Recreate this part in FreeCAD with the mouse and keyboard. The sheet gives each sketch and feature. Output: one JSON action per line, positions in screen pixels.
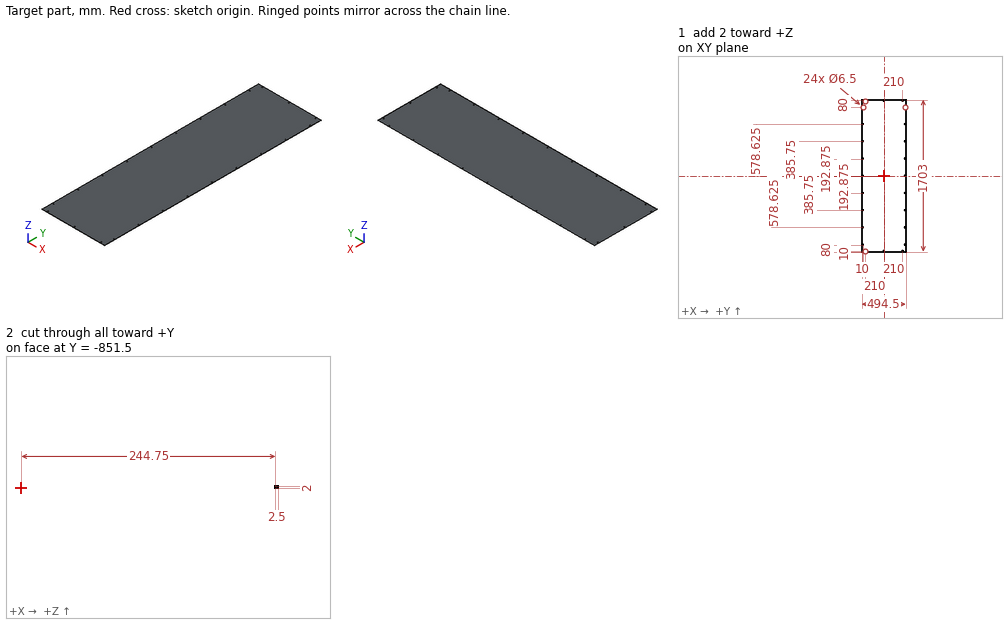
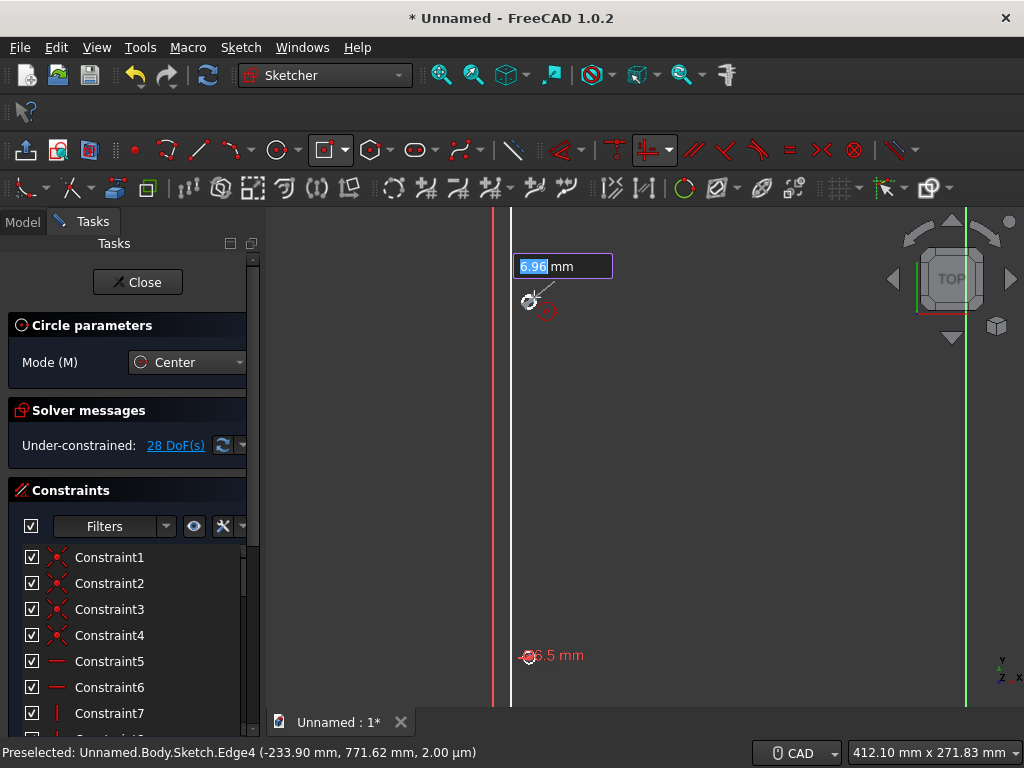
{"action": "type", "text": "6.5"}
{"action": "key", "text": "Return"}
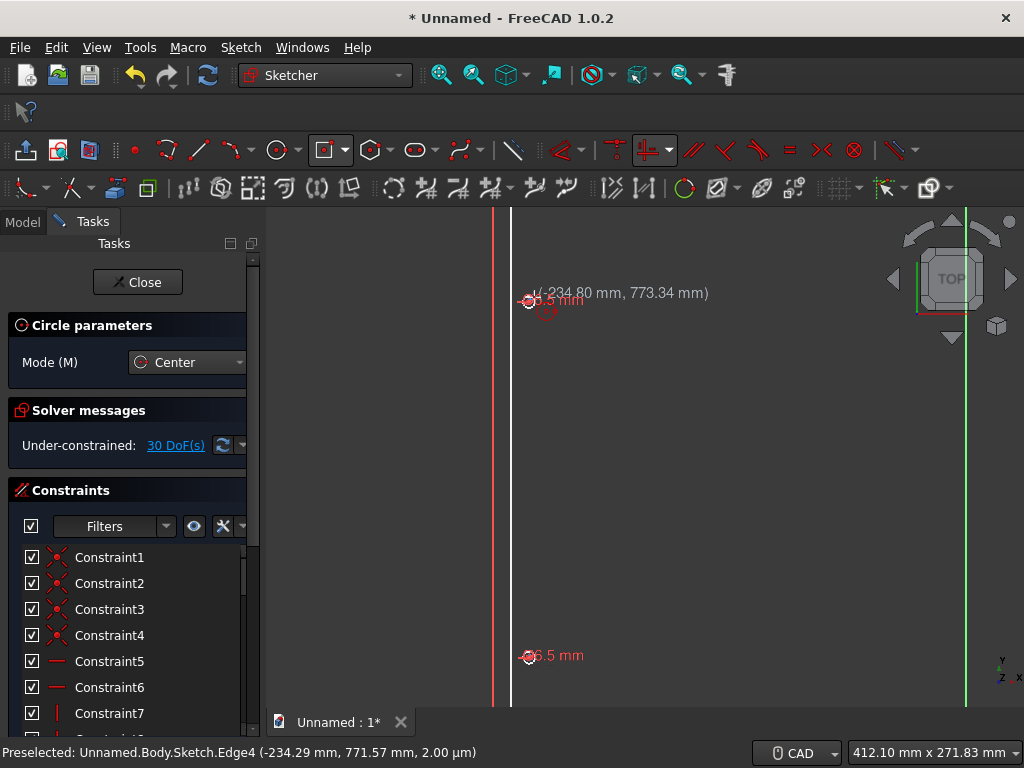
{"action": "scroll", "coordinate": [538, 331], "scroll_direction": "down", "scroll_amount": 12}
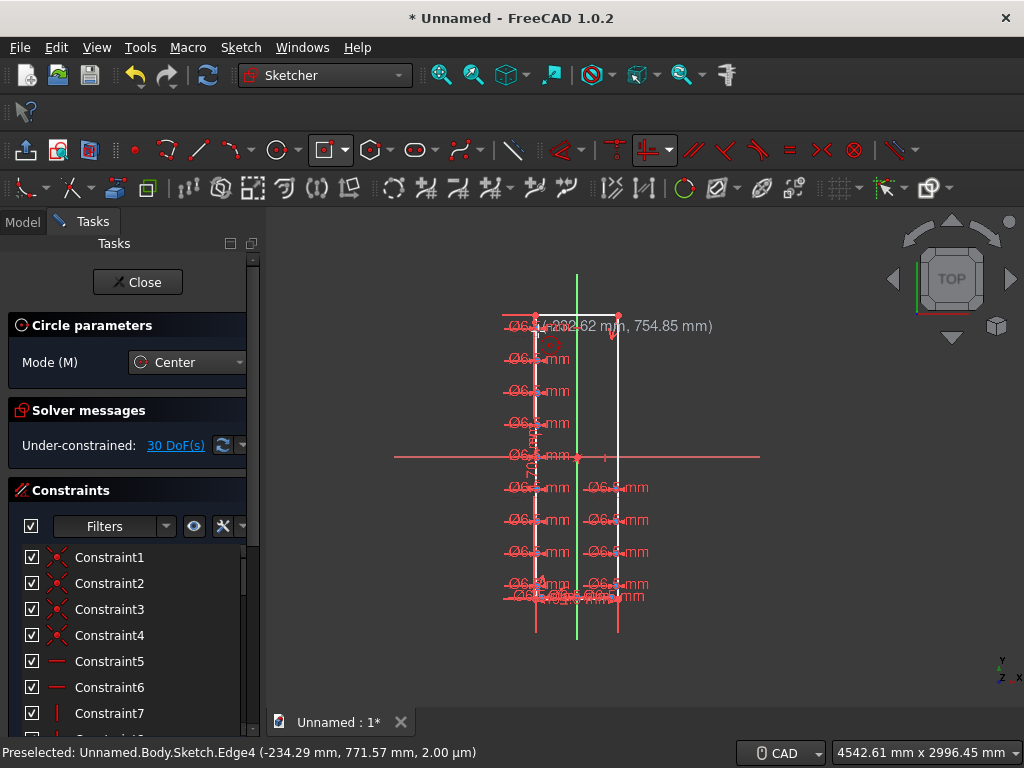
{"action": "scroll", "coordinate": [542, 317], "scroll_direction": "up", "scroll_amount": 19}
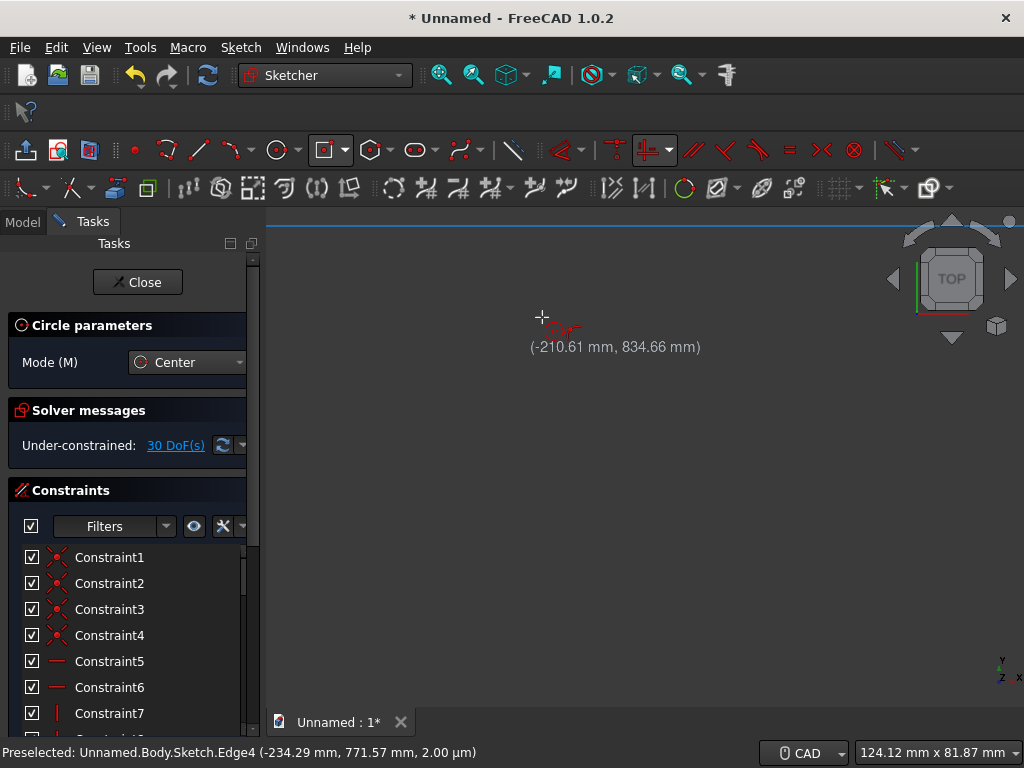
{"action": "scroll", "coordinate": [534, 285], "scroll_direction": "down", "scroll_amount": 18}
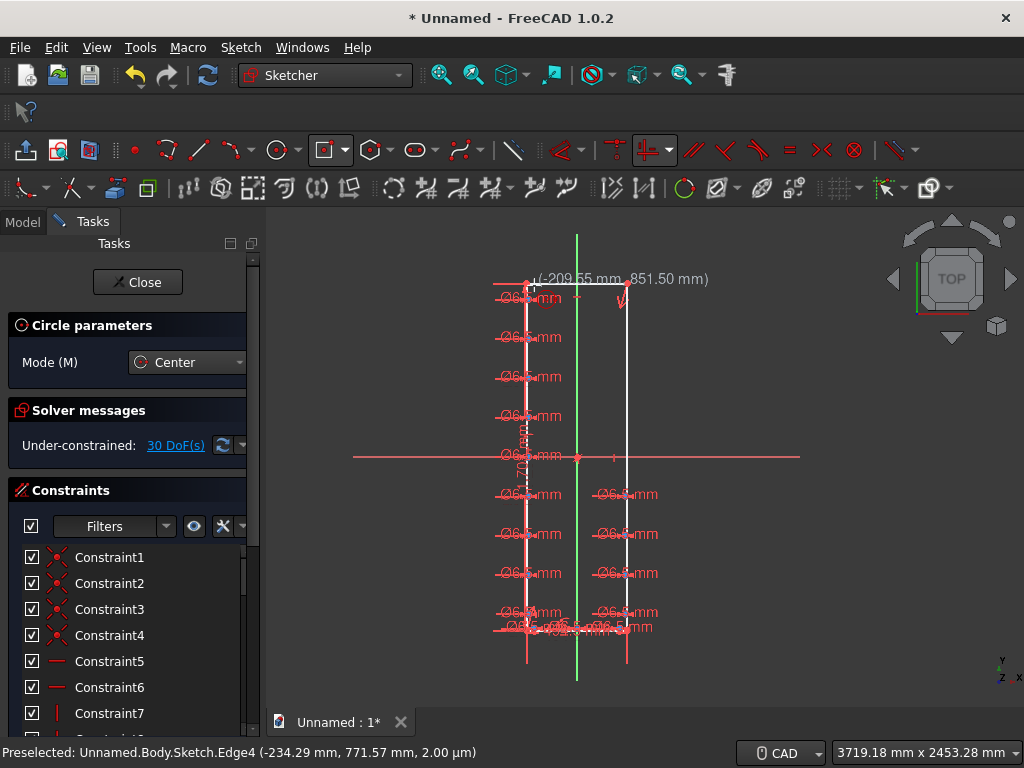
{"action": "scroll", "coordinate": [534, 286], "scroll_direction": "up", "scroll_amount": 11}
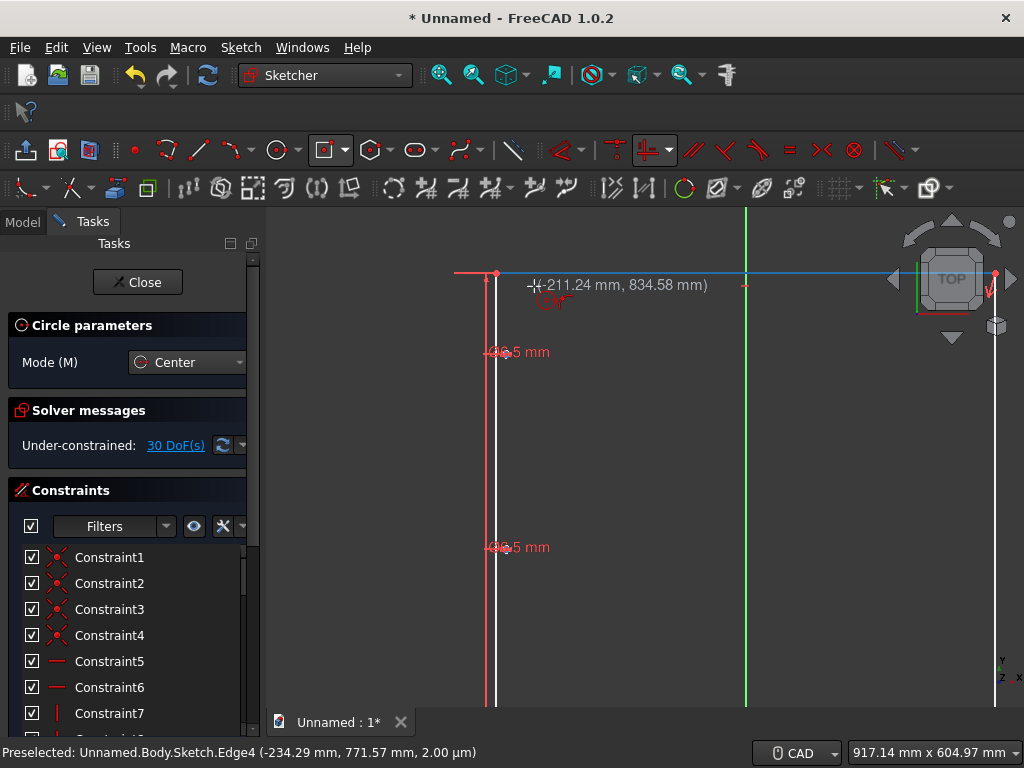
{"action": "left_click", "coordinate": [533, 281]}
{"action": "mouse_move", "coordinate": [538, 277]}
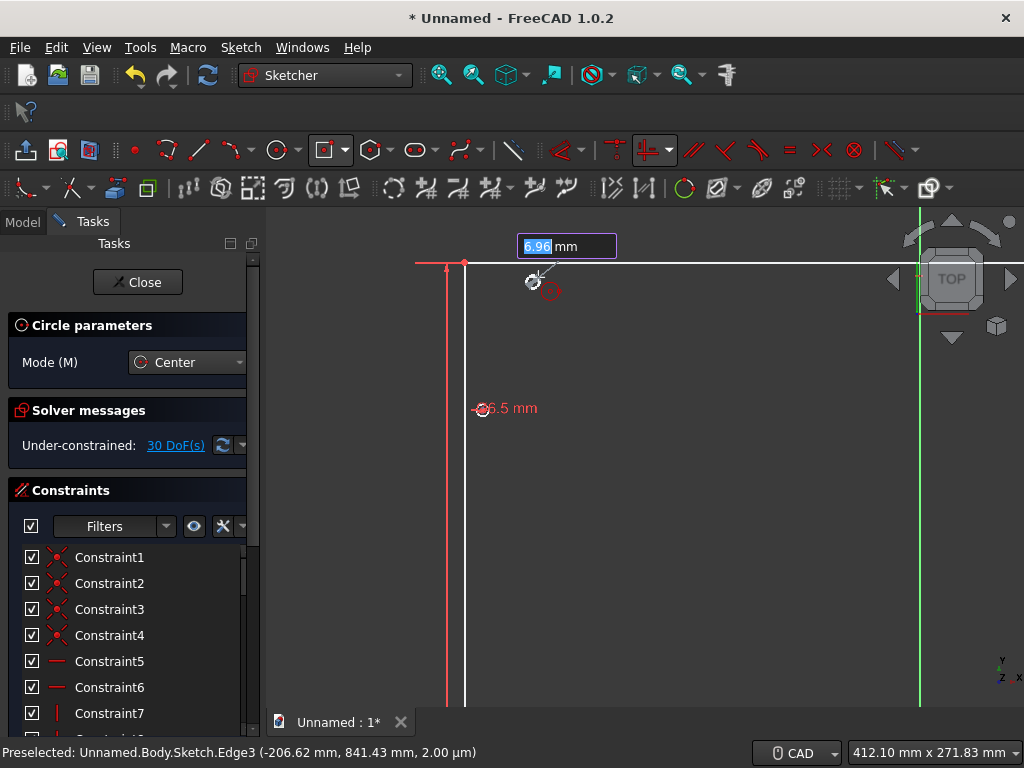
{"action": "type", "text": "6.5"}
{"action": "key", "text": "Return"}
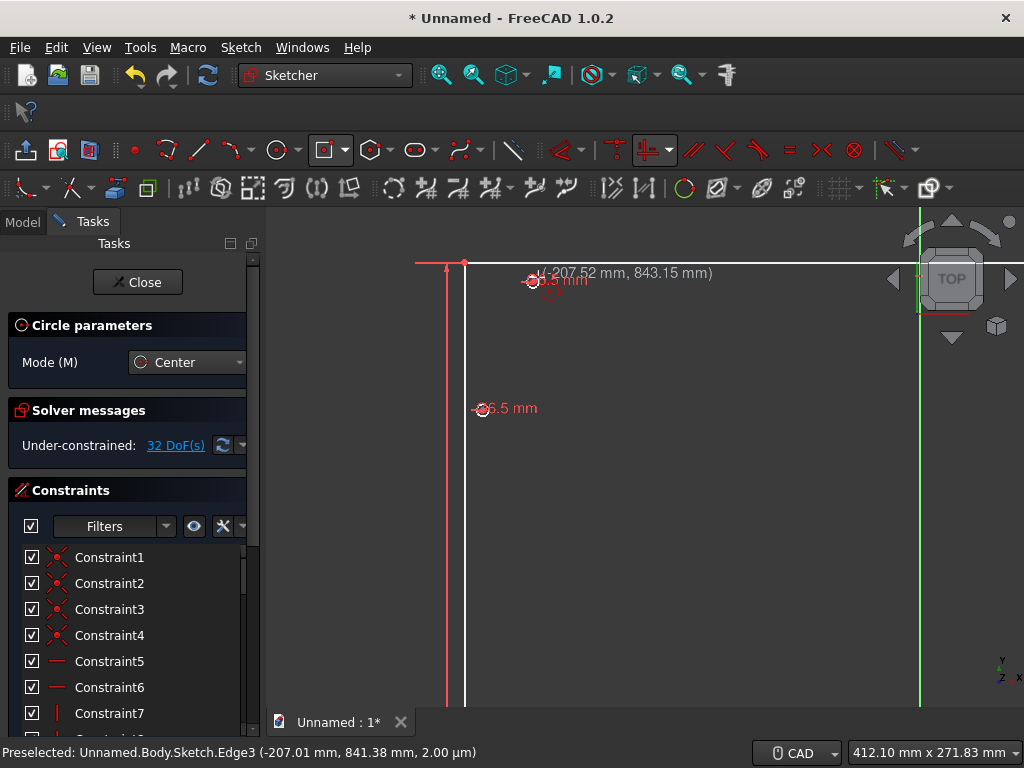
{"action": "scroll", "coordinate": [542, 320], "scroll_direction": "down", "scroll_amount": 12}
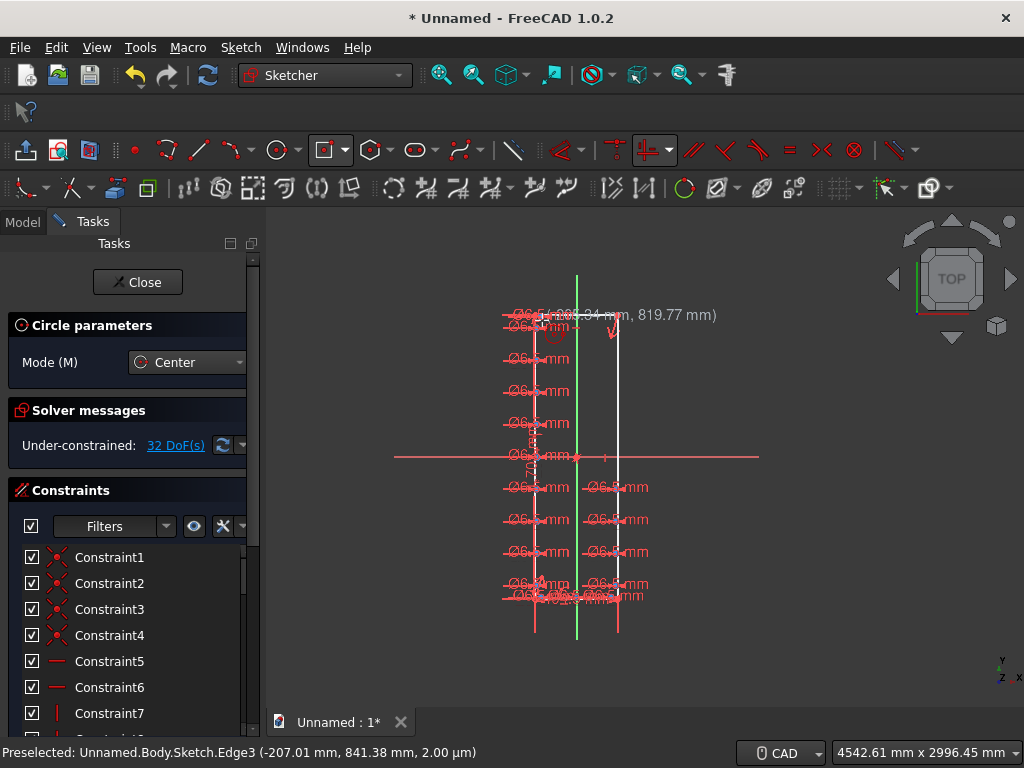
{"action": "scroll", "coordinate": [616, 457], "scroll_direction": "up", "scroll_amount": 19}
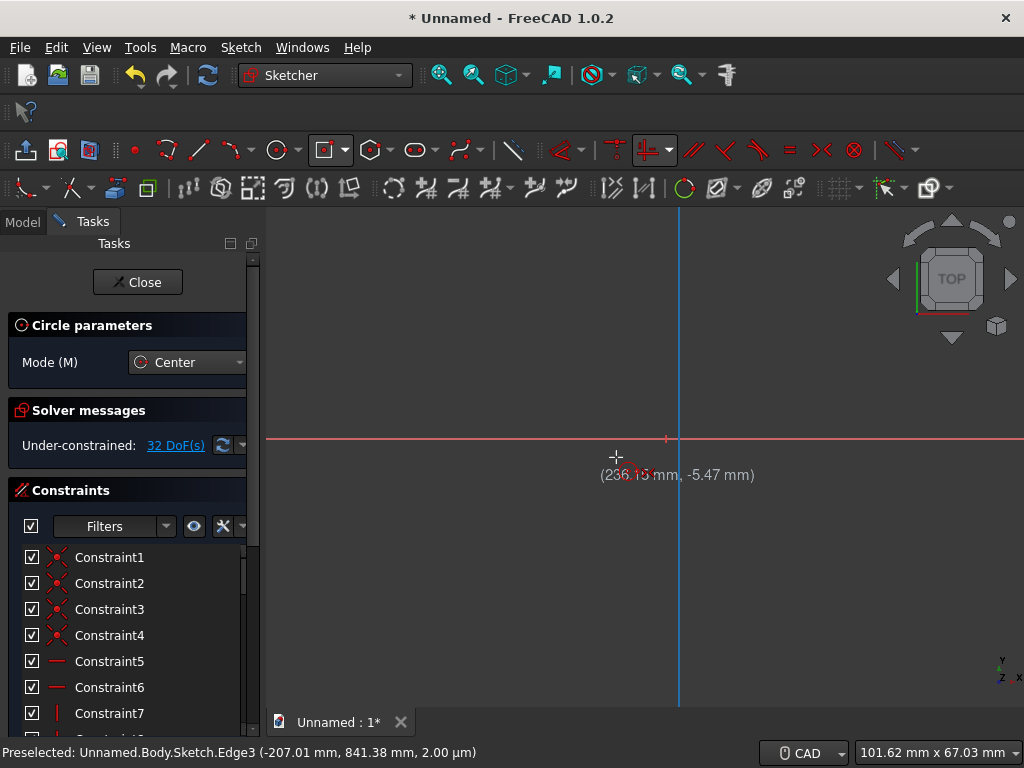
{"action": "scroll", "coordinate": [625, 458], "scroll_direction": "down", "scroll_amount": 18}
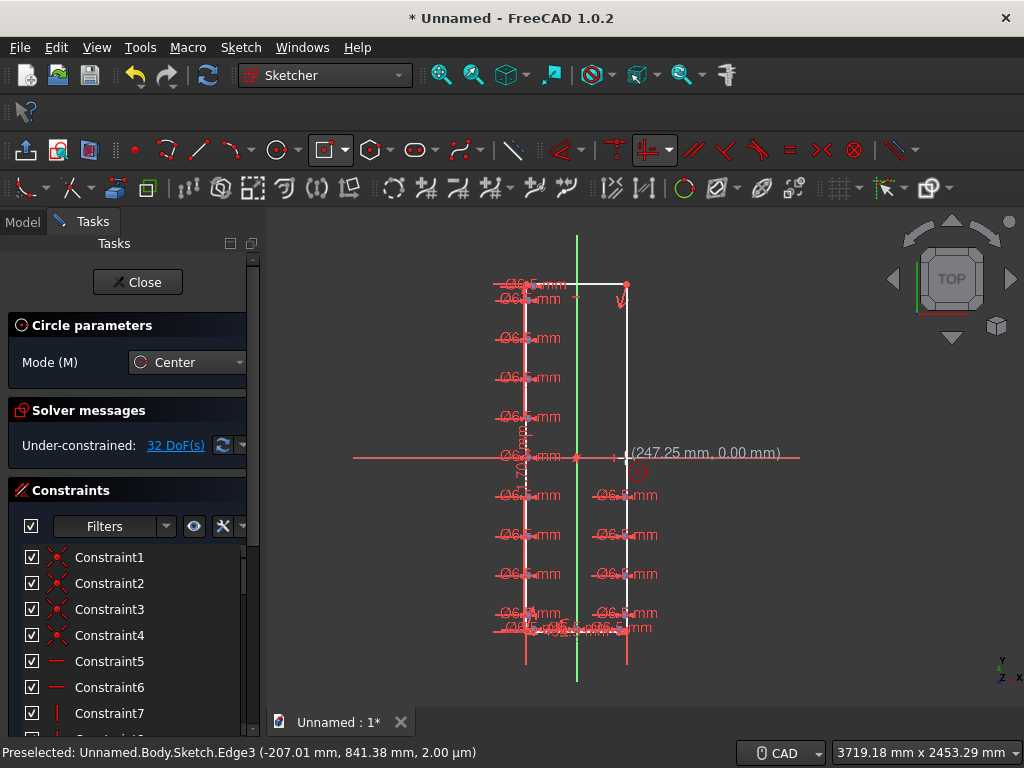
{"action": "scroll", "coordinate": [625, 458], "scroll_direction": "up", "scroll_amount": 11}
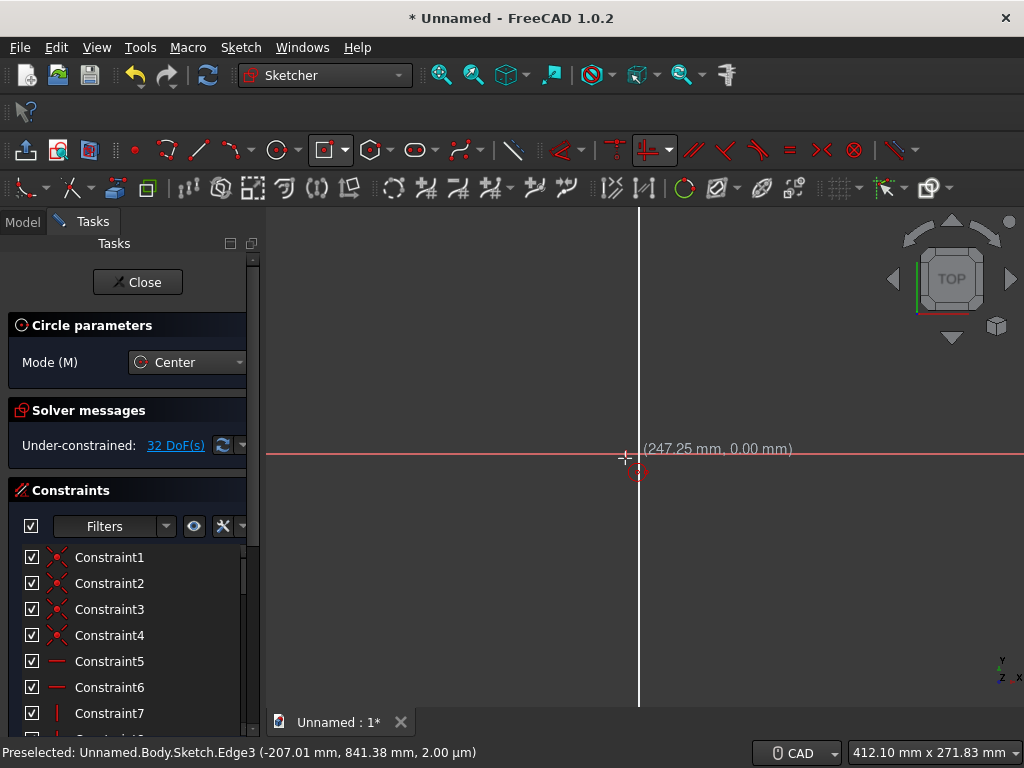
{"action": "left_click", "coordinate": [620, 454]}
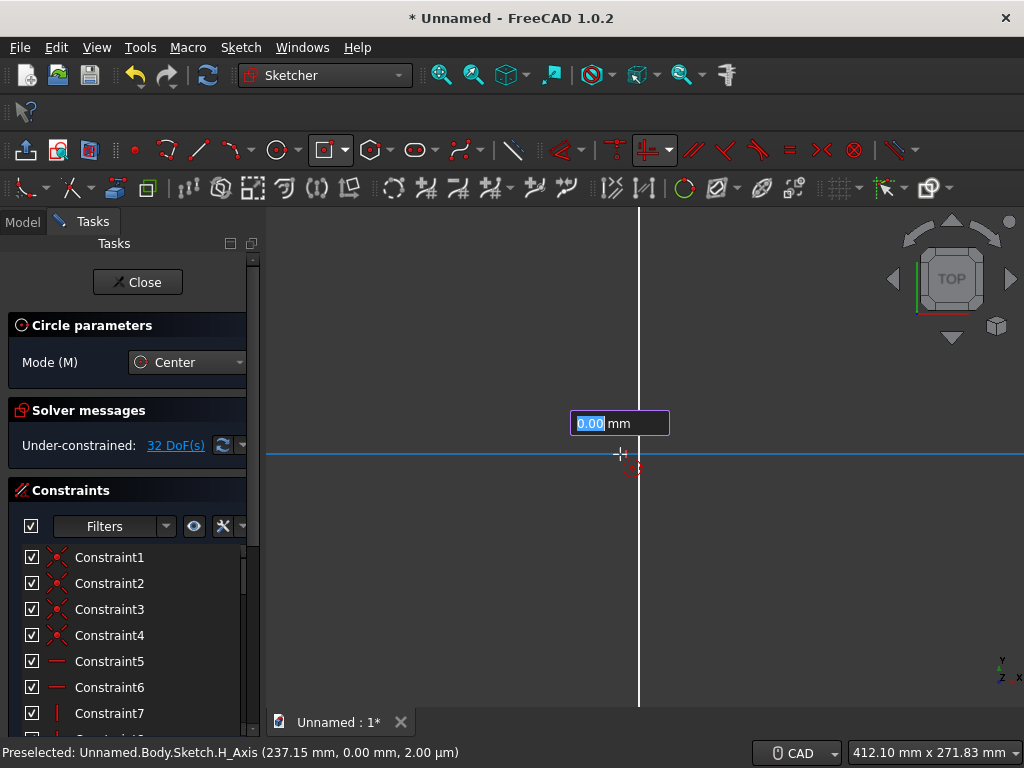
{"action": "scroll", "coordinate": [618, 459], "scroll_direction": "up", "scroll_amount": 6}
{"action": "mouse_move", "coordinate": [617, 459]}